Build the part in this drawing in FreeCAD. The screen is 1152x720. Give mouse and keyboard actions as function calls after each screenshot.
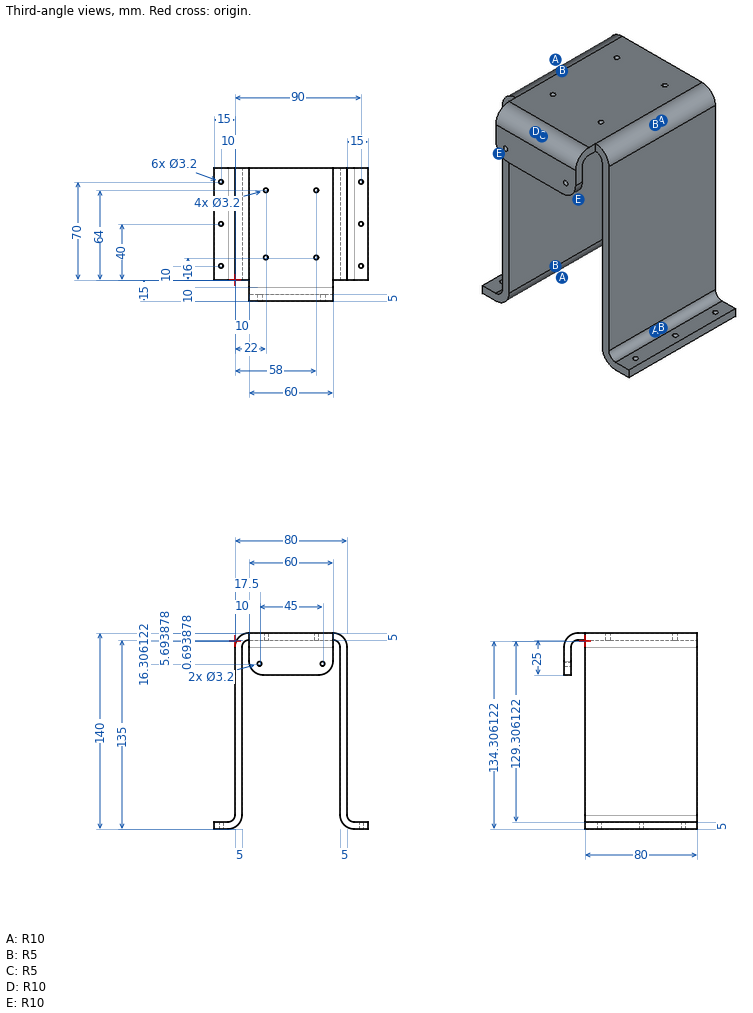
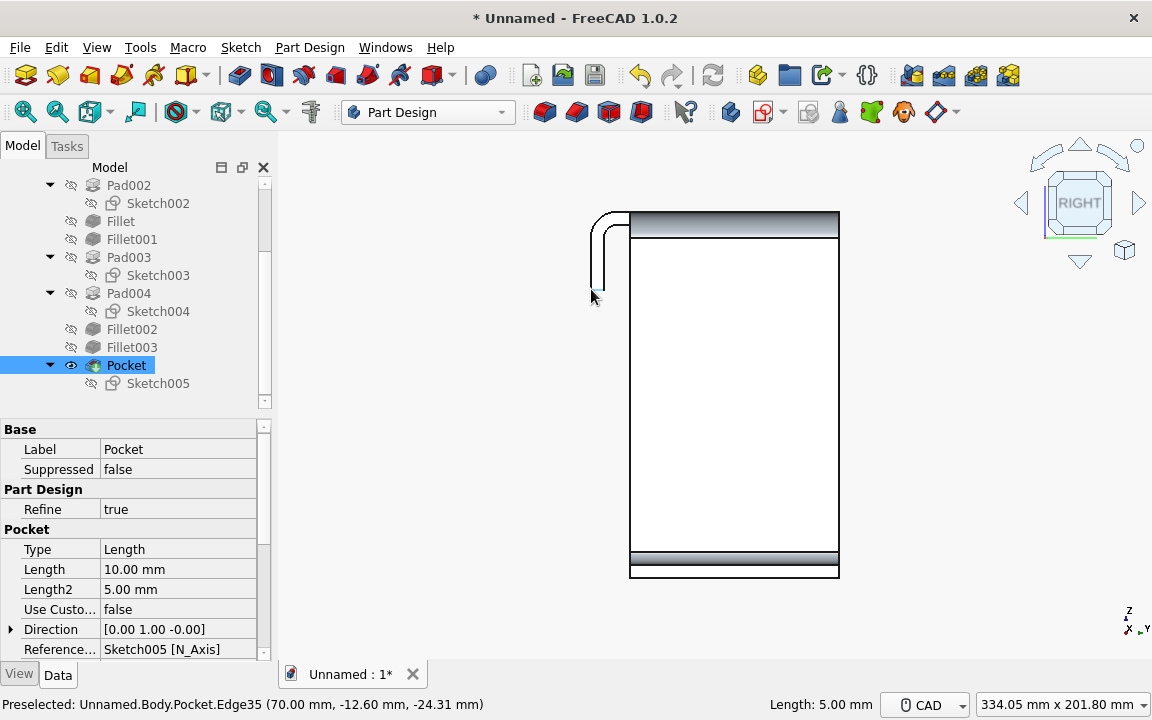
scroll(597, 289, up, 6)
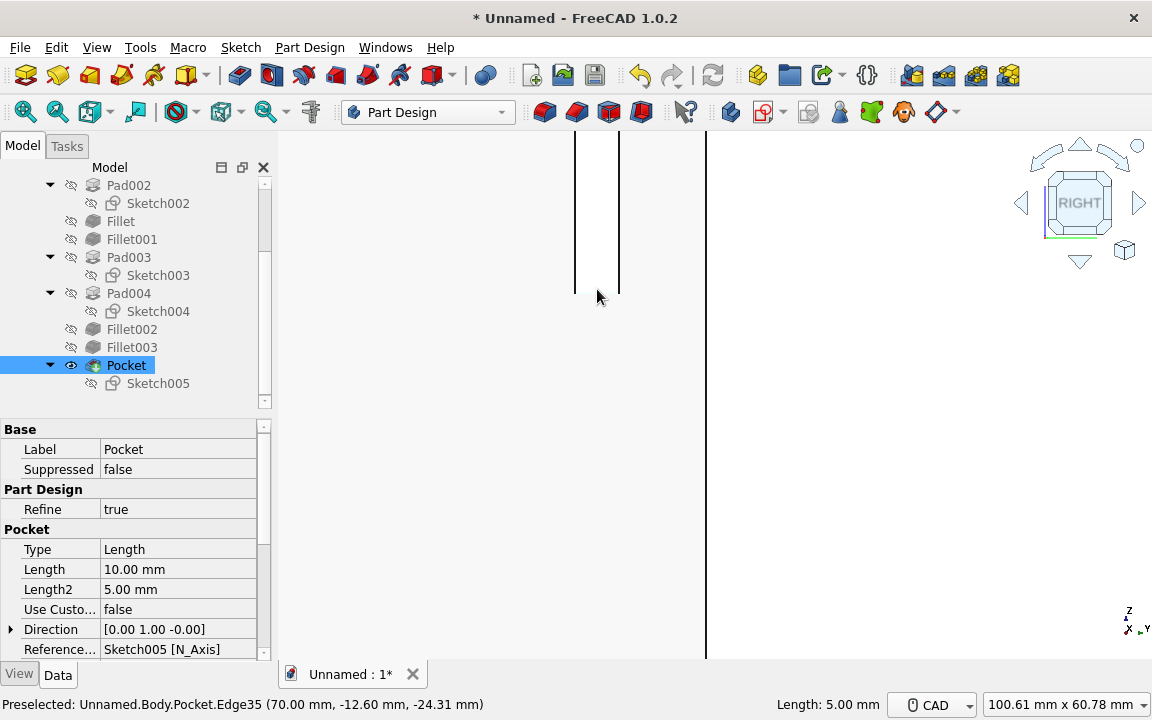
key(v)
key(f)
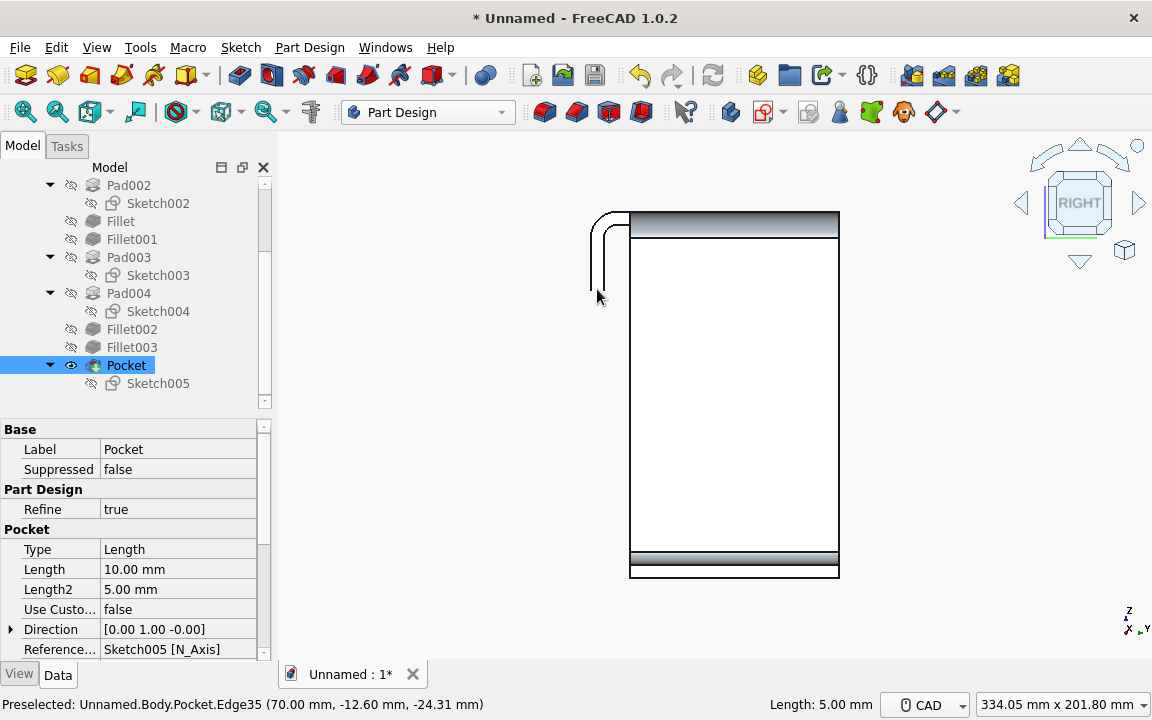
key(5)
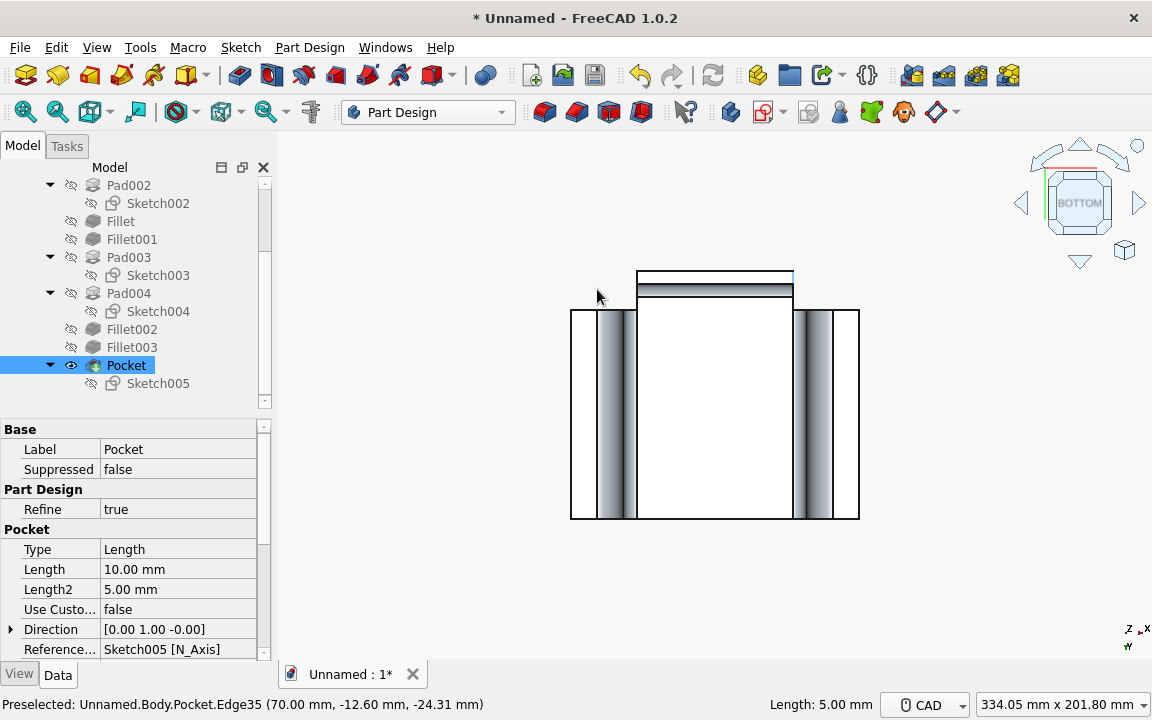
click(637, 276, ctrl)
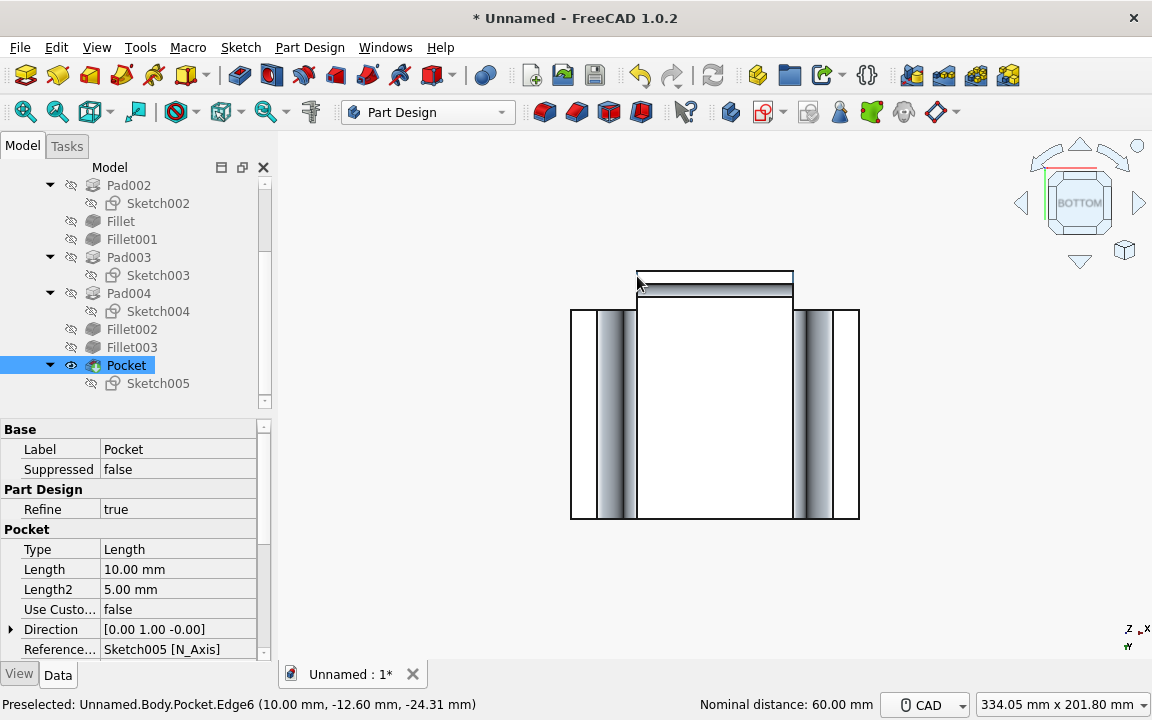
click(546, 112)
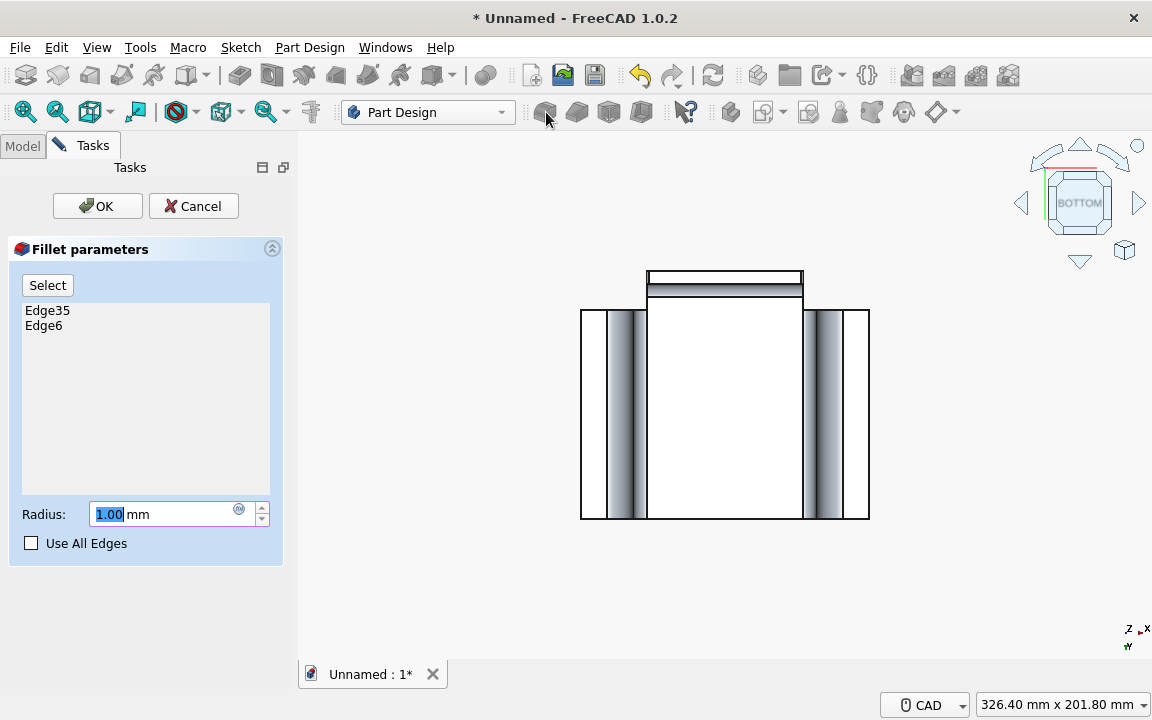
text(10)
key(Tab)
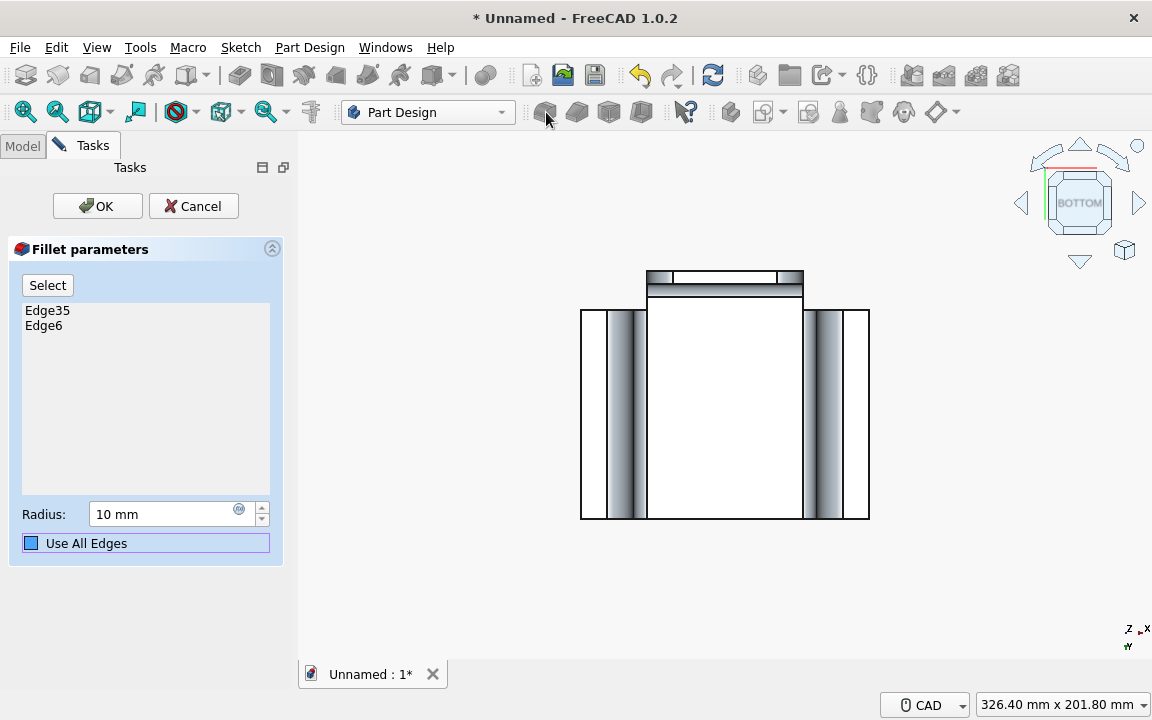
click(98, 206)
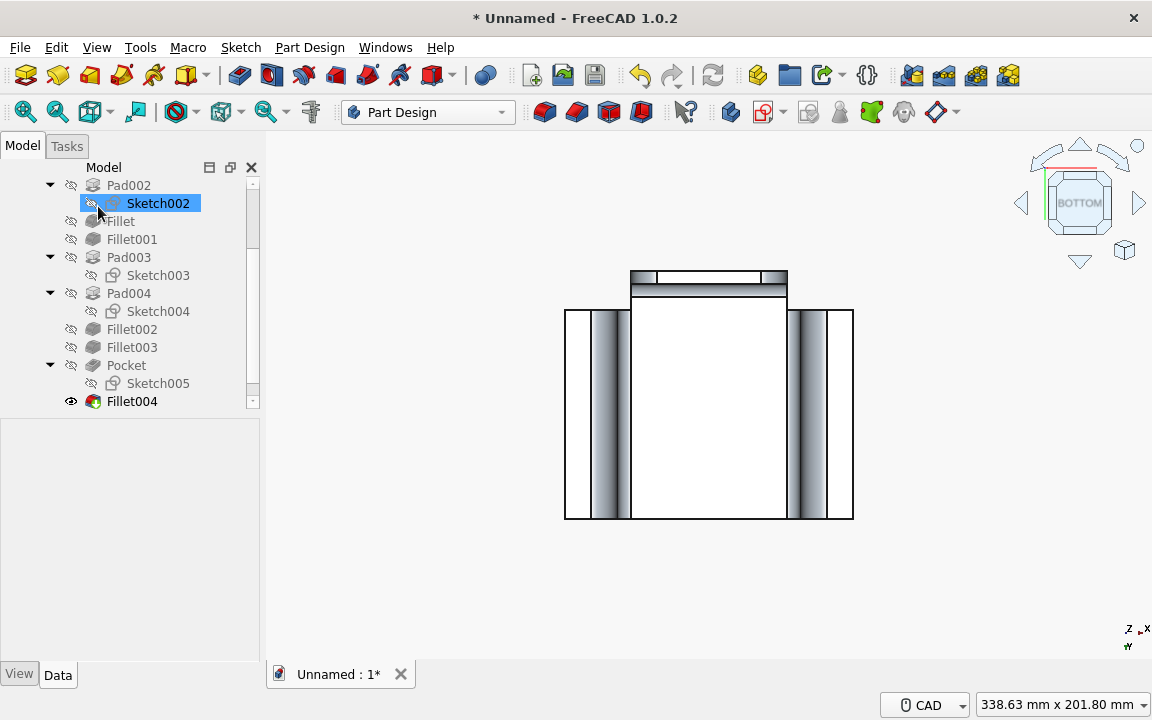
key(0)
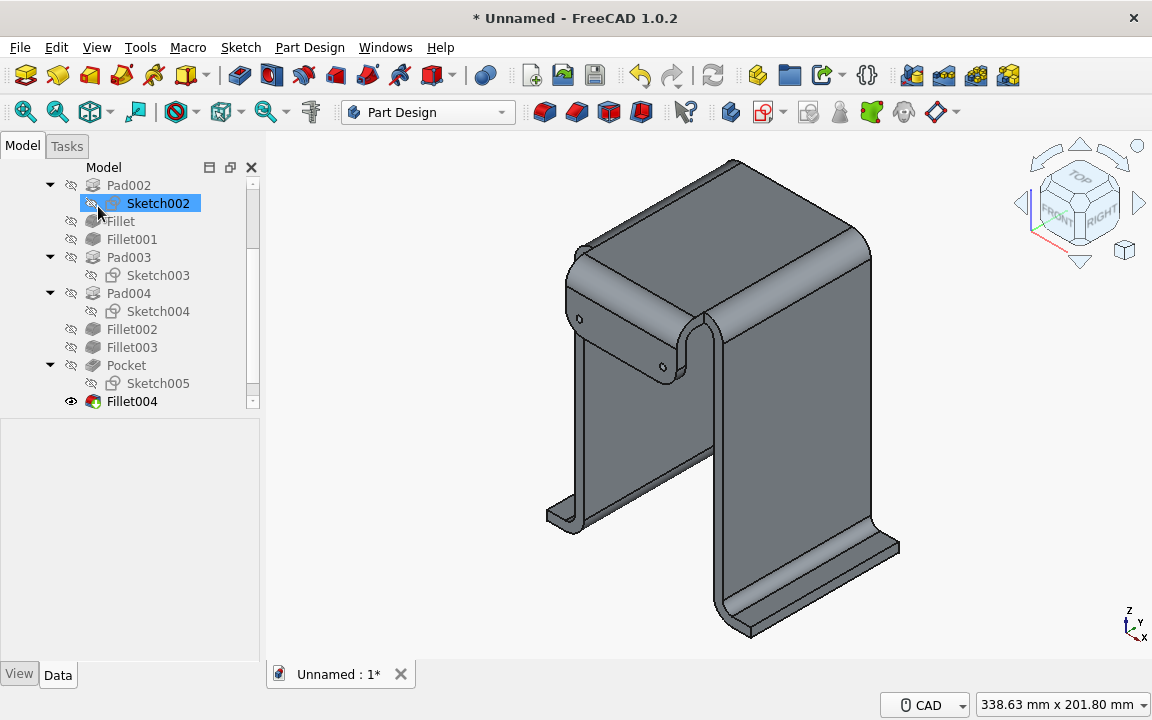
click(741, 226)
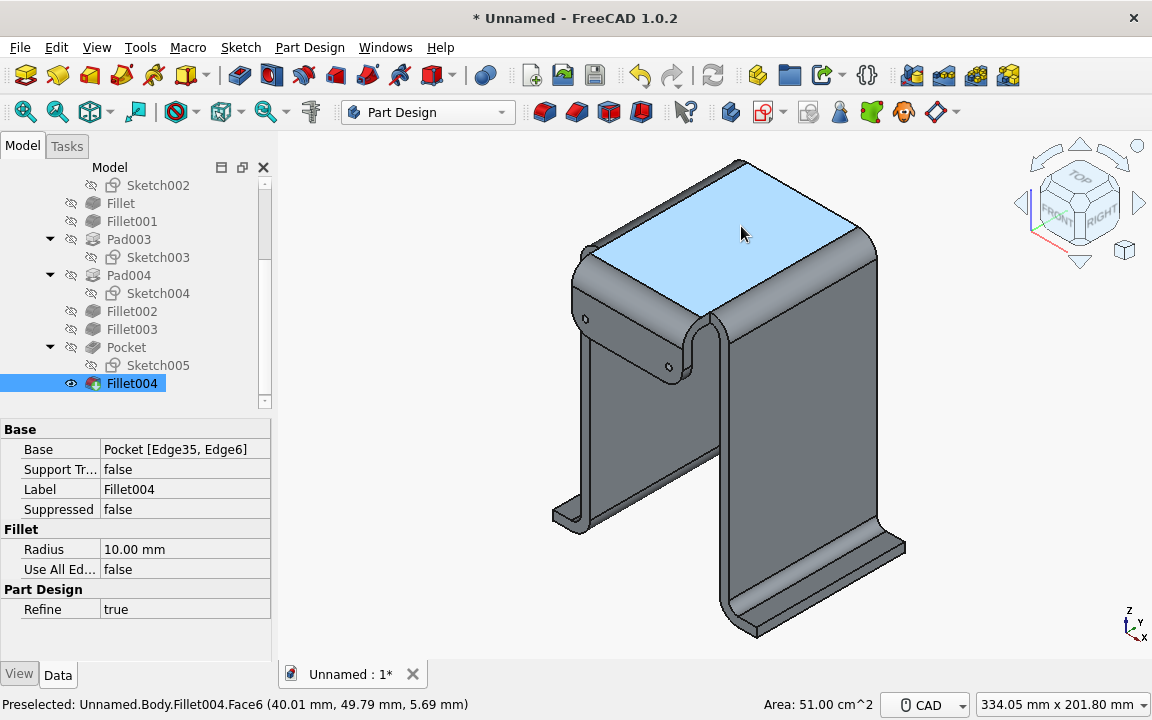
click(764, 112)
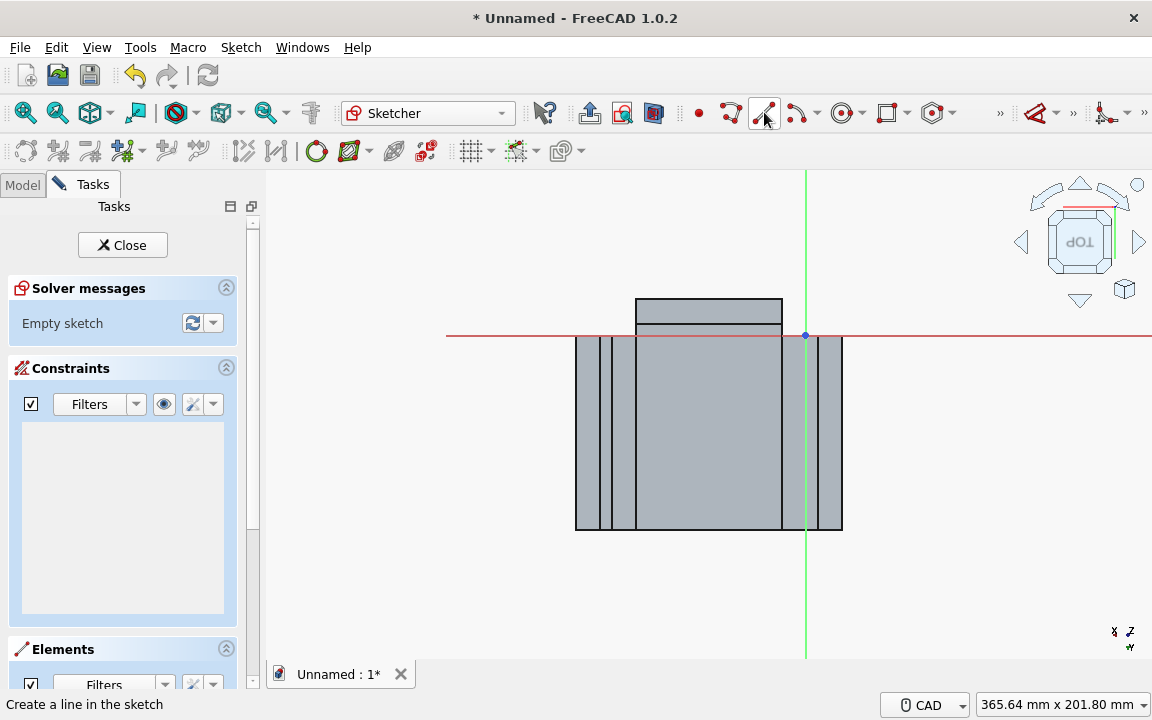
scroll(847, 416, up, 3)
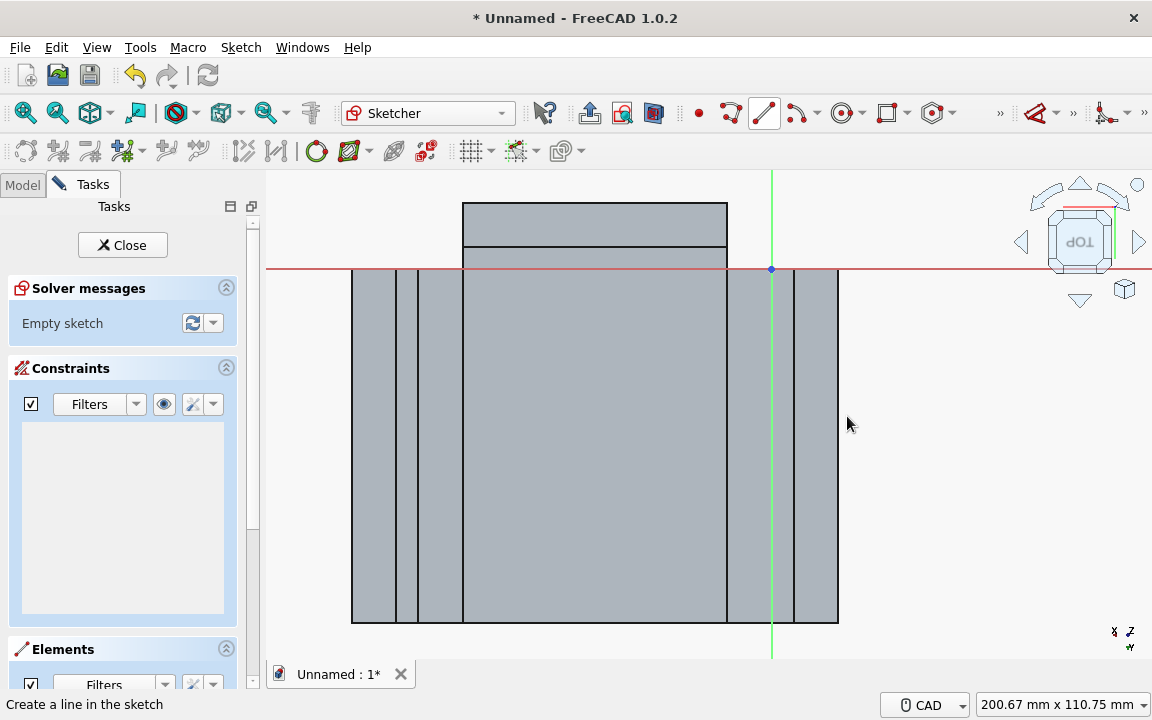
click(842, 114)